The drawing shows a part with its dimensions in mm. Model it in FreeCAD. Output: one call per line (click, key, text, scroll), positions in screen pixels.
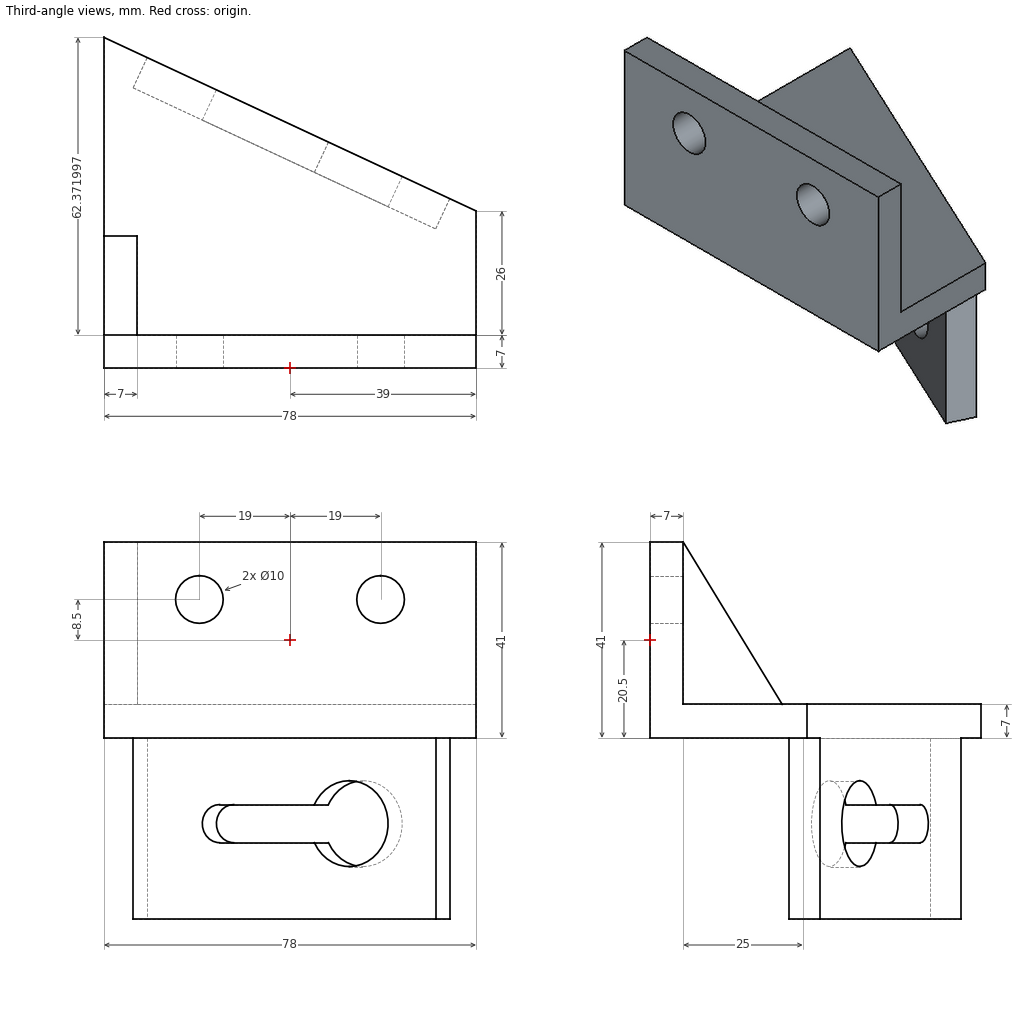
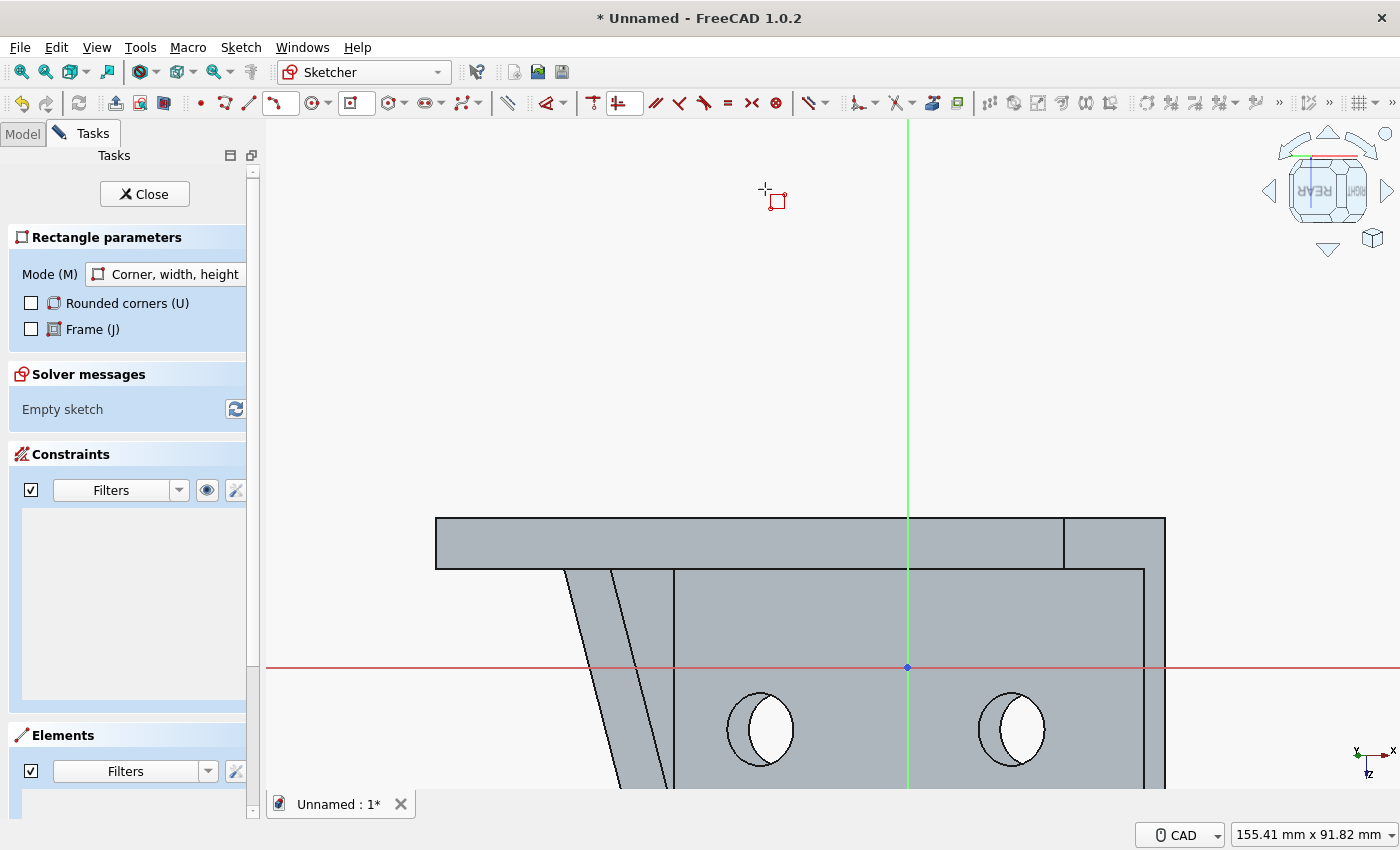
click(509, 241)
move(1019, 518)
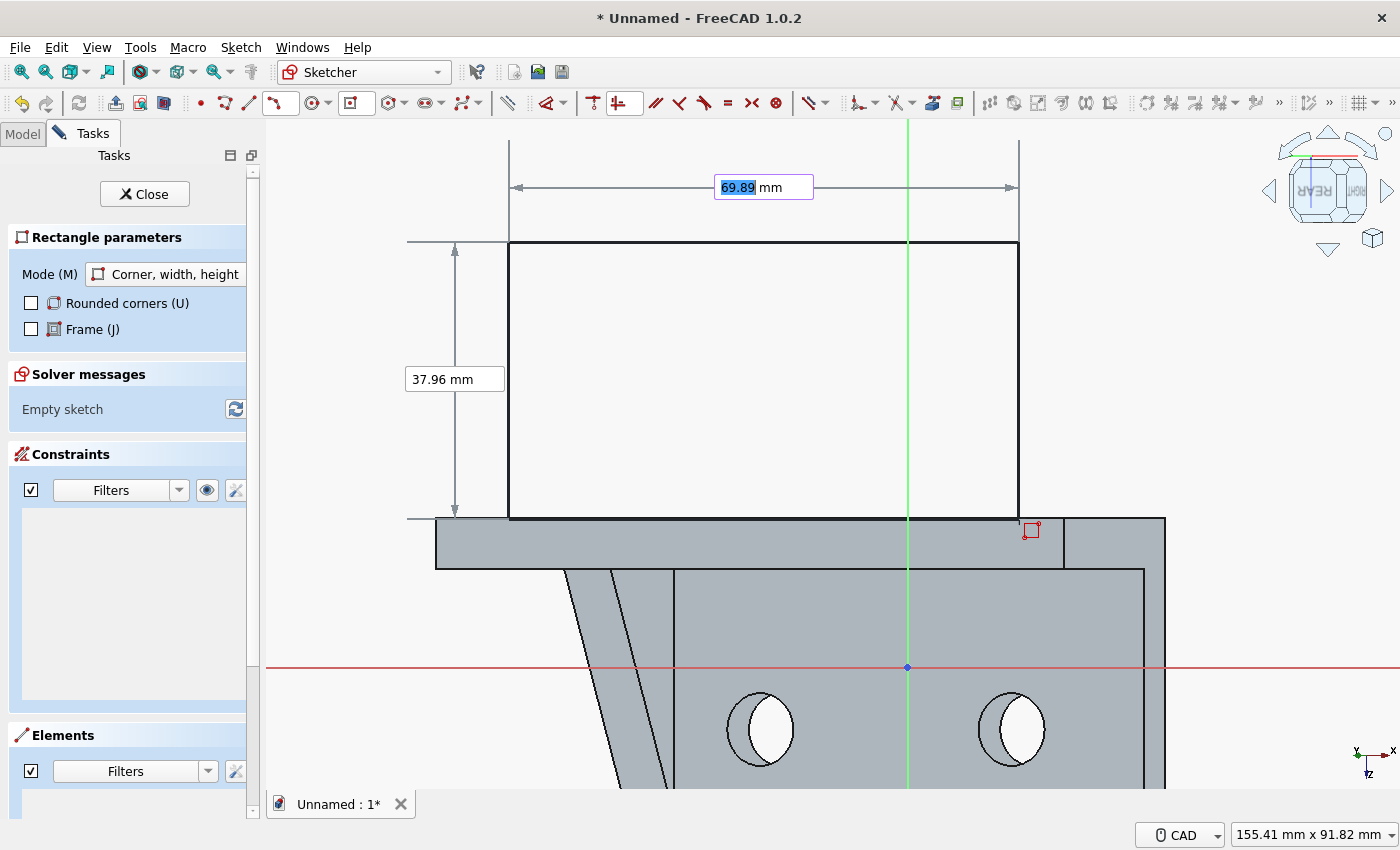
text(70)
key(Tab)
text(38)
key(Return)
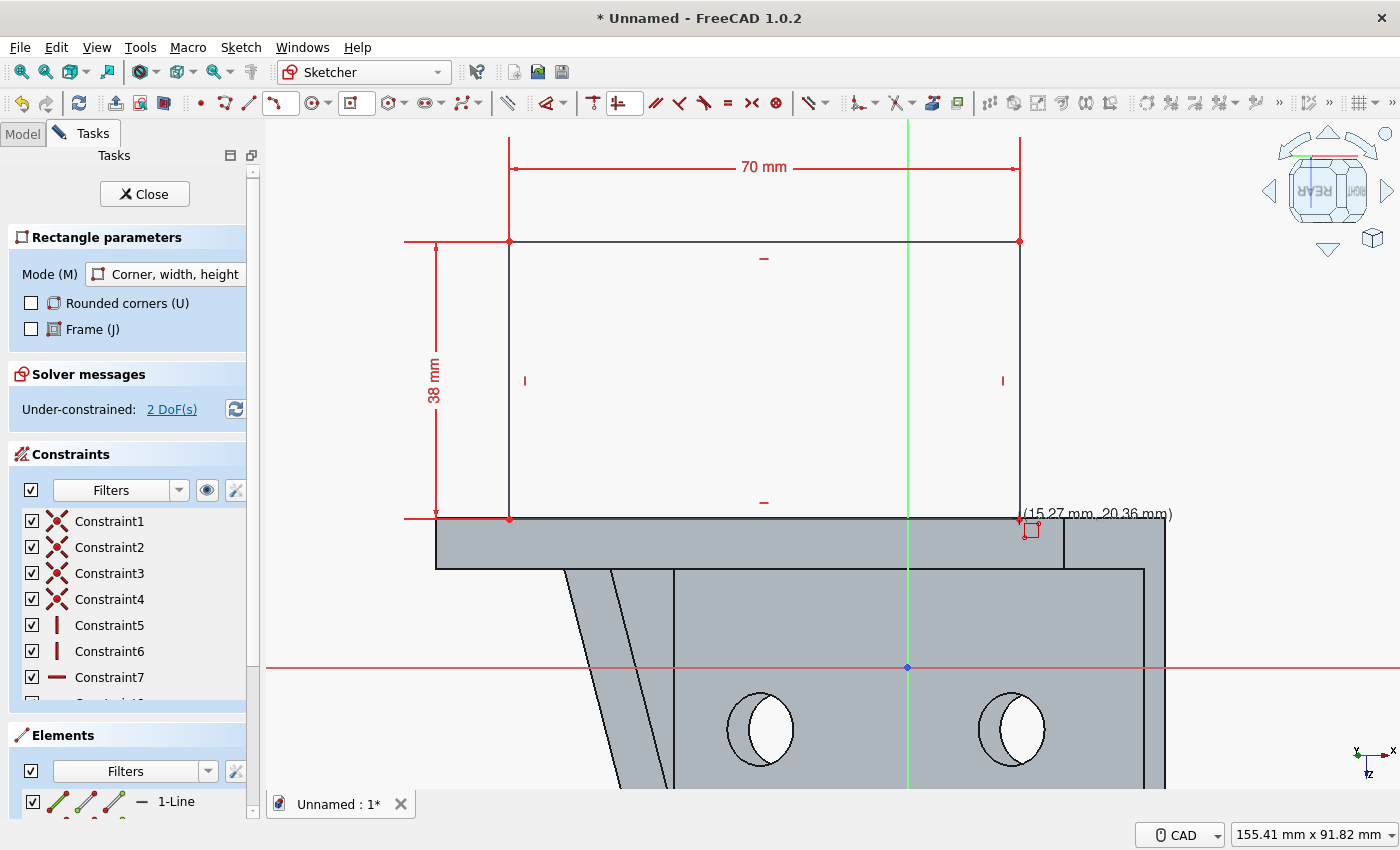
click(250, 104)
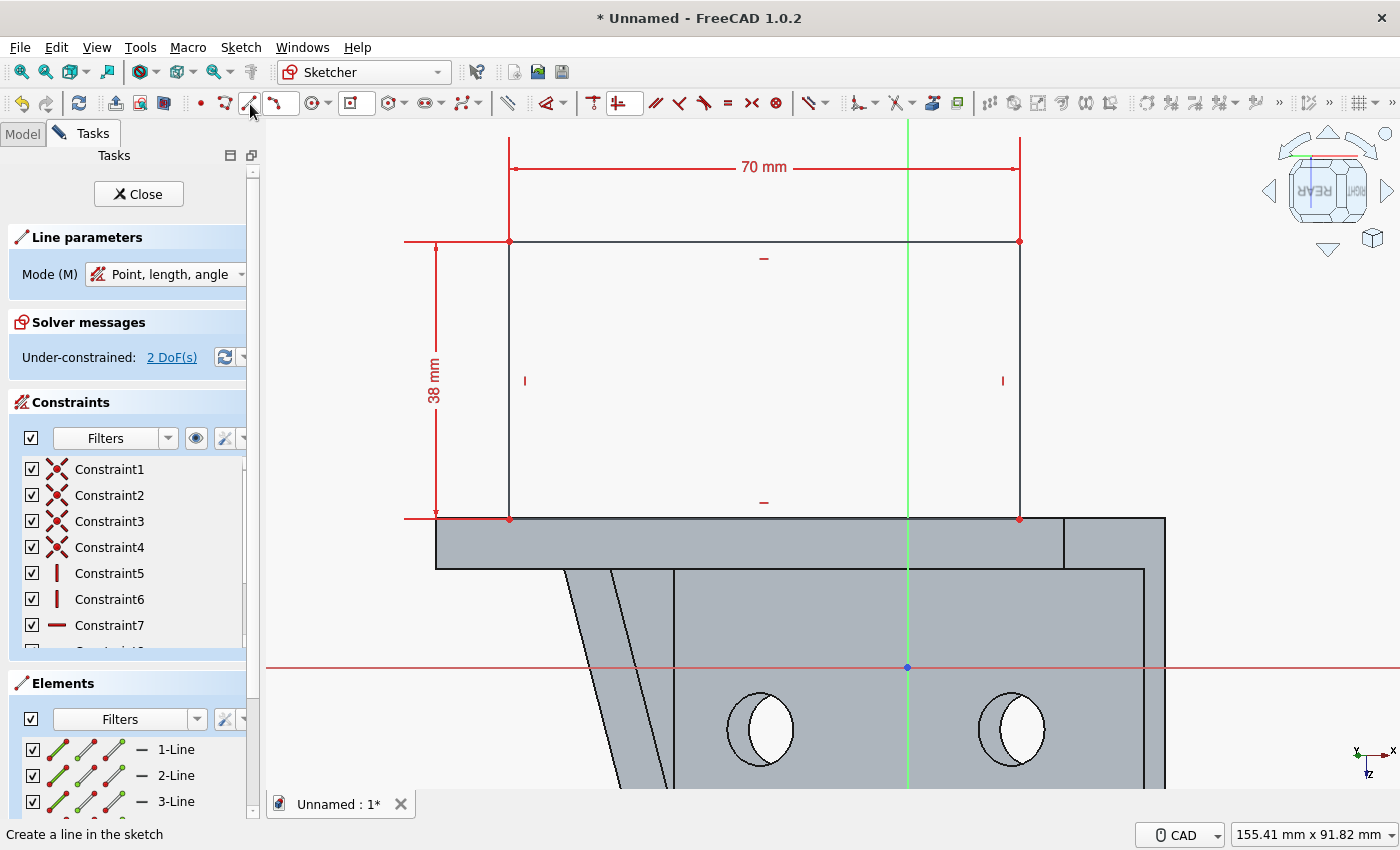
click(655, 357)
click(815, 357)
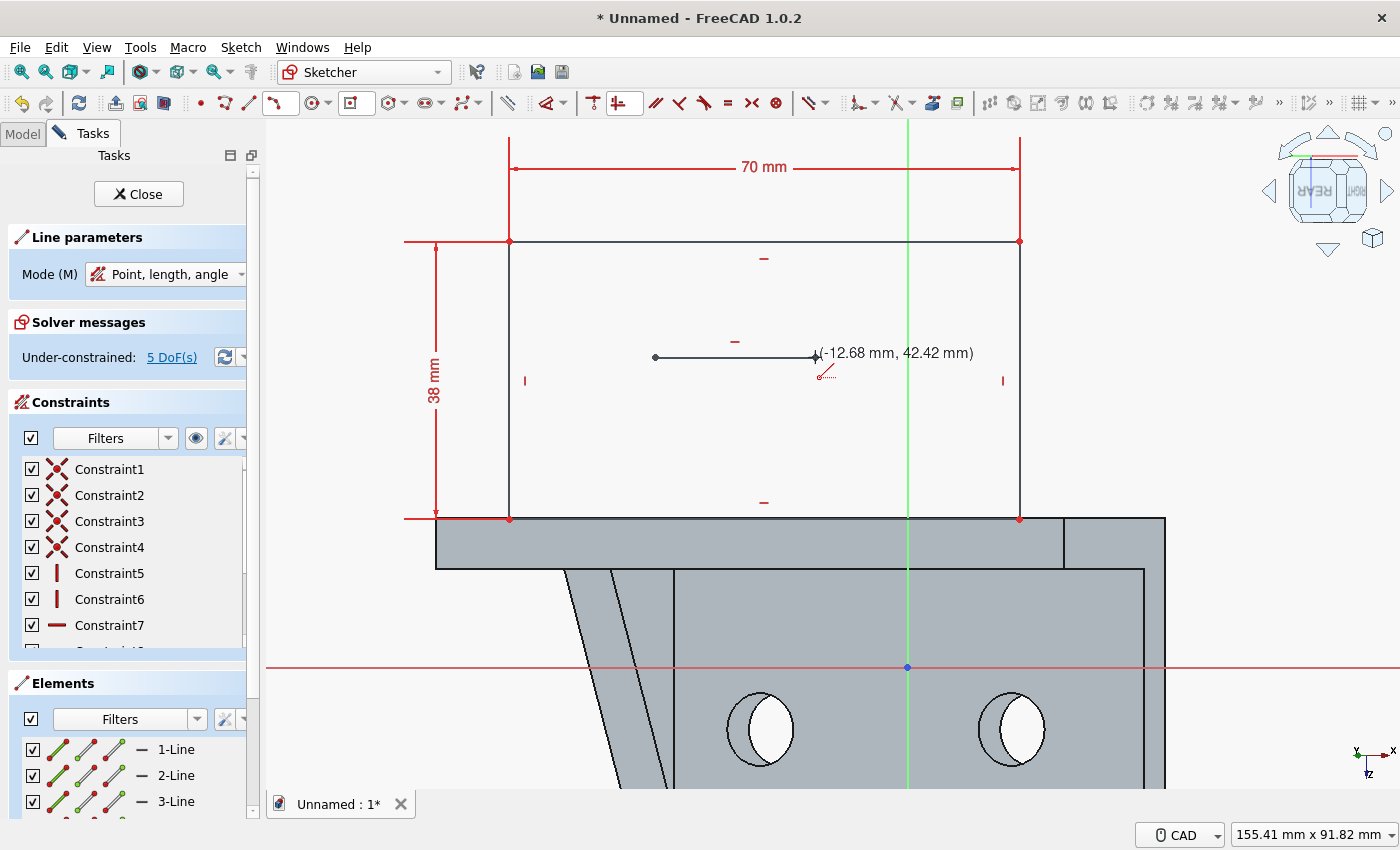
click(815, 416)
click(655, 416)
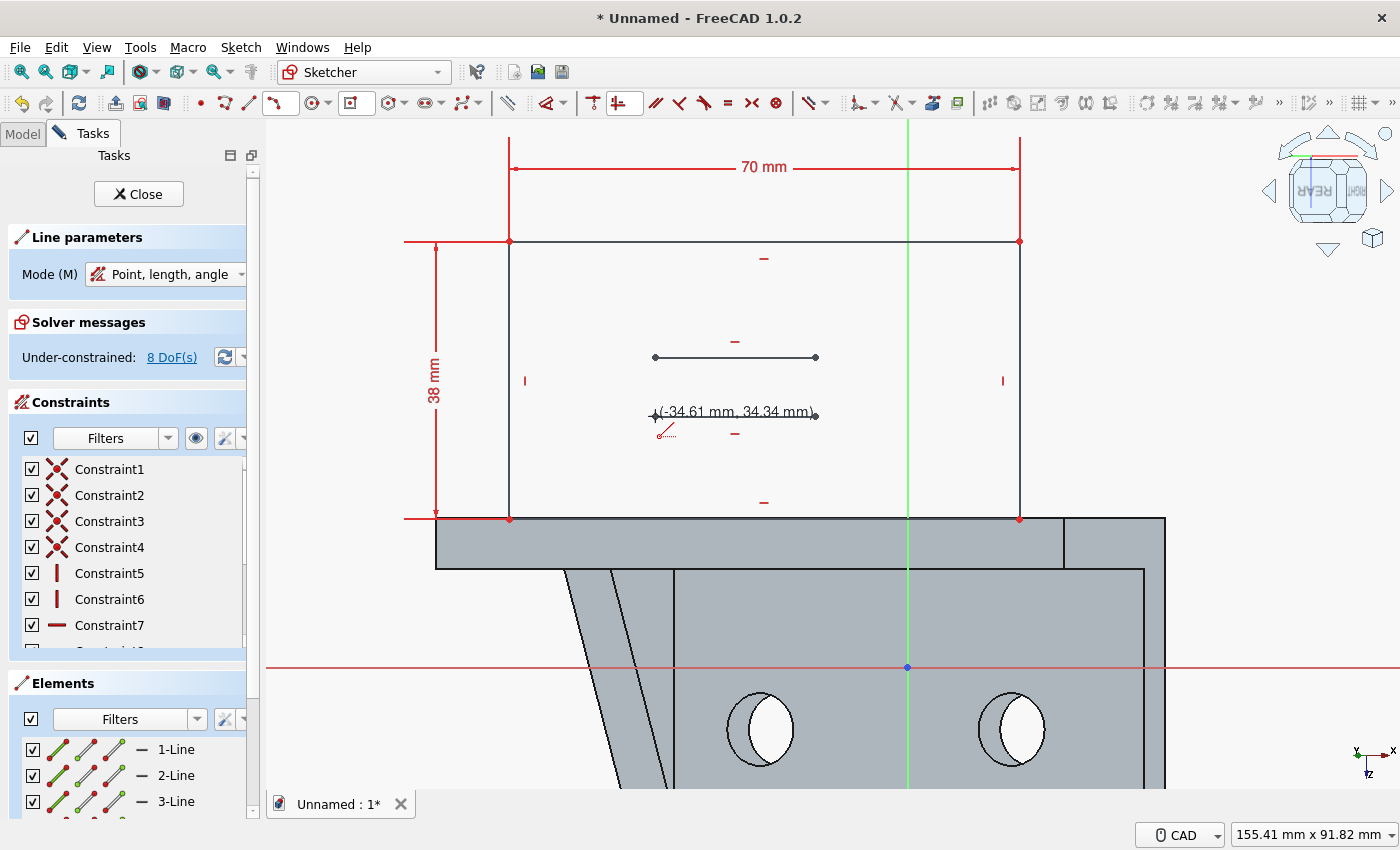
click(274, 104)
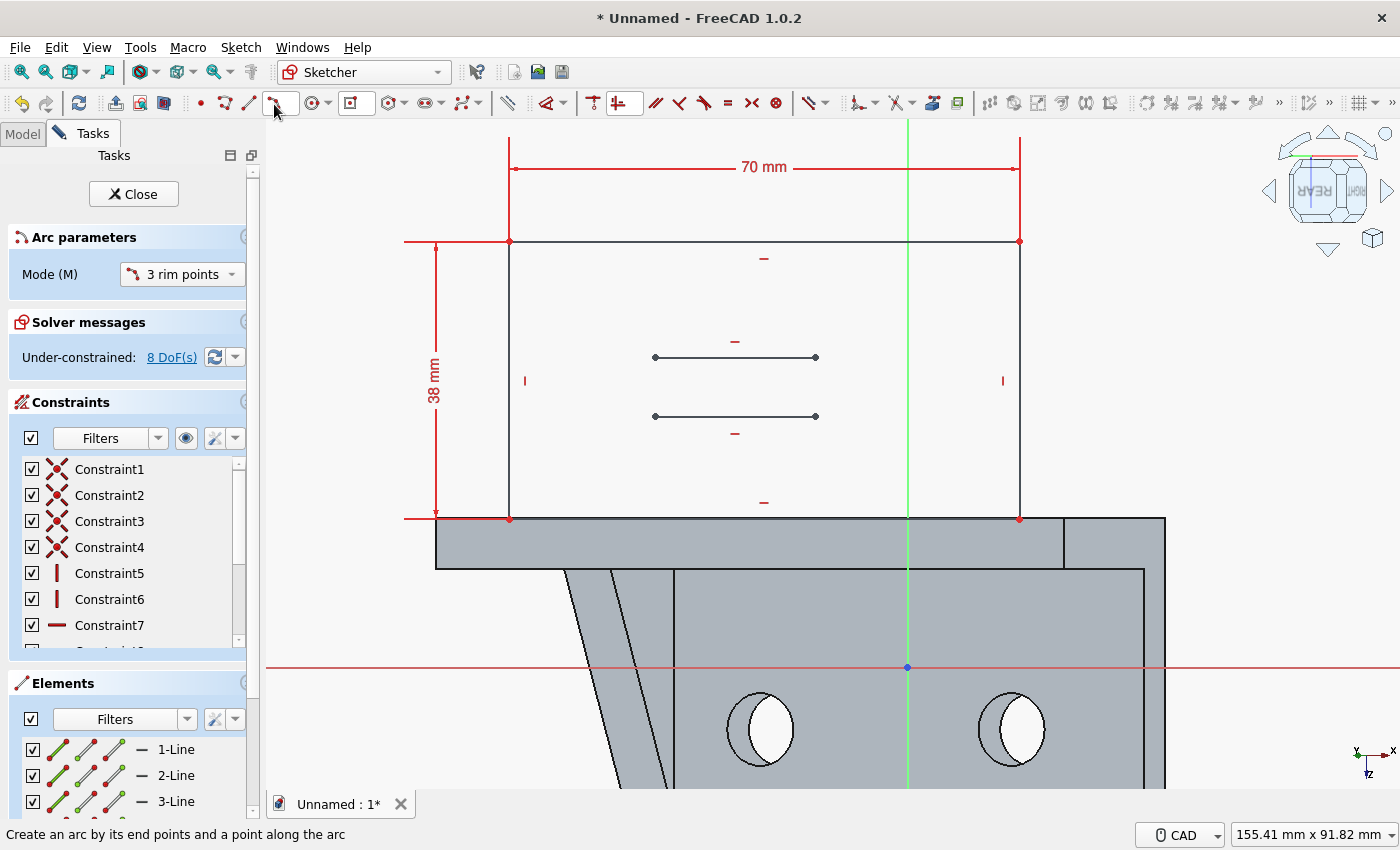
click(815, 358)
click(815, 417)
click(939, 387)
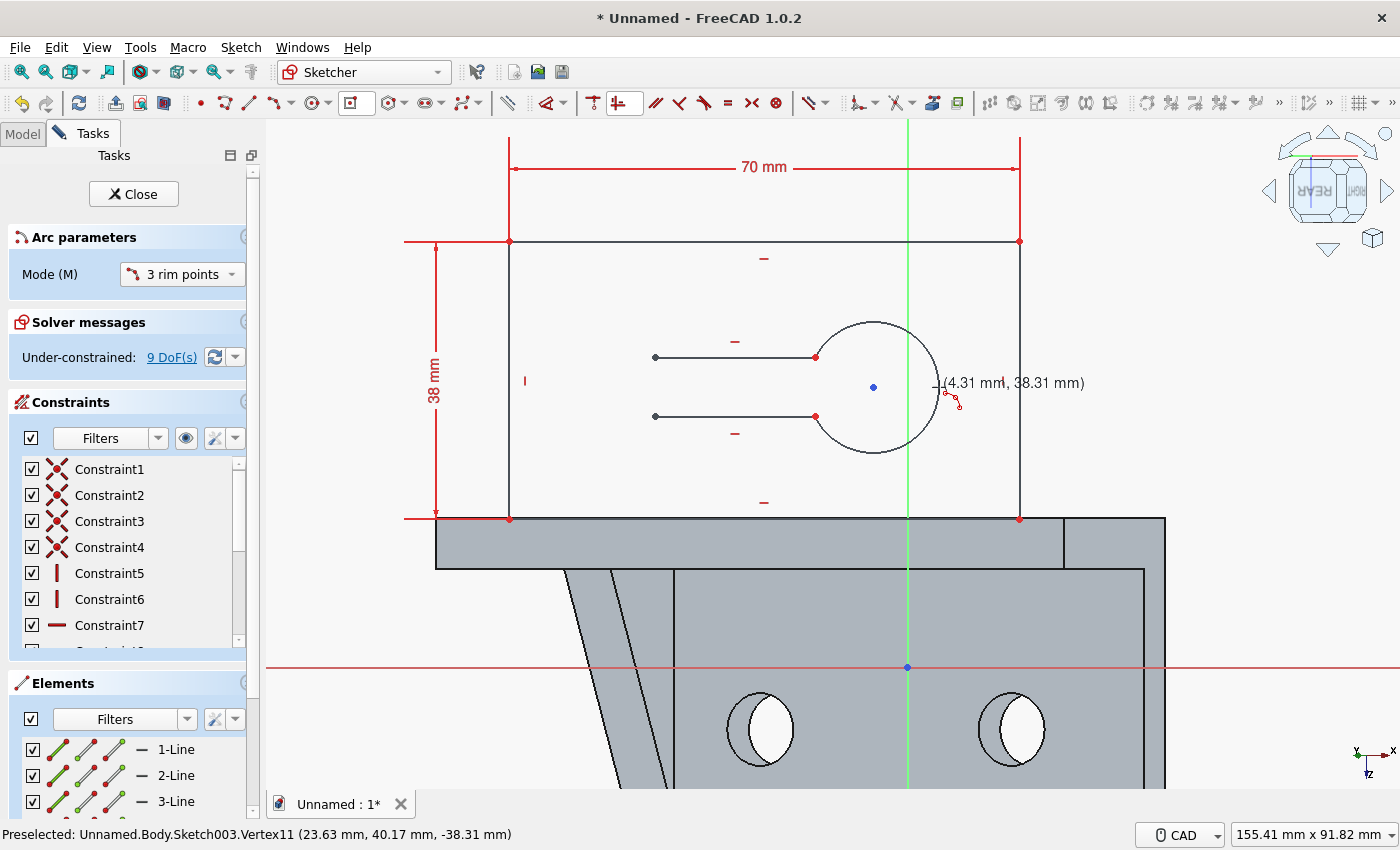
click(655, 417)
click(655, 358)
click(625, 387)
key(Escape)